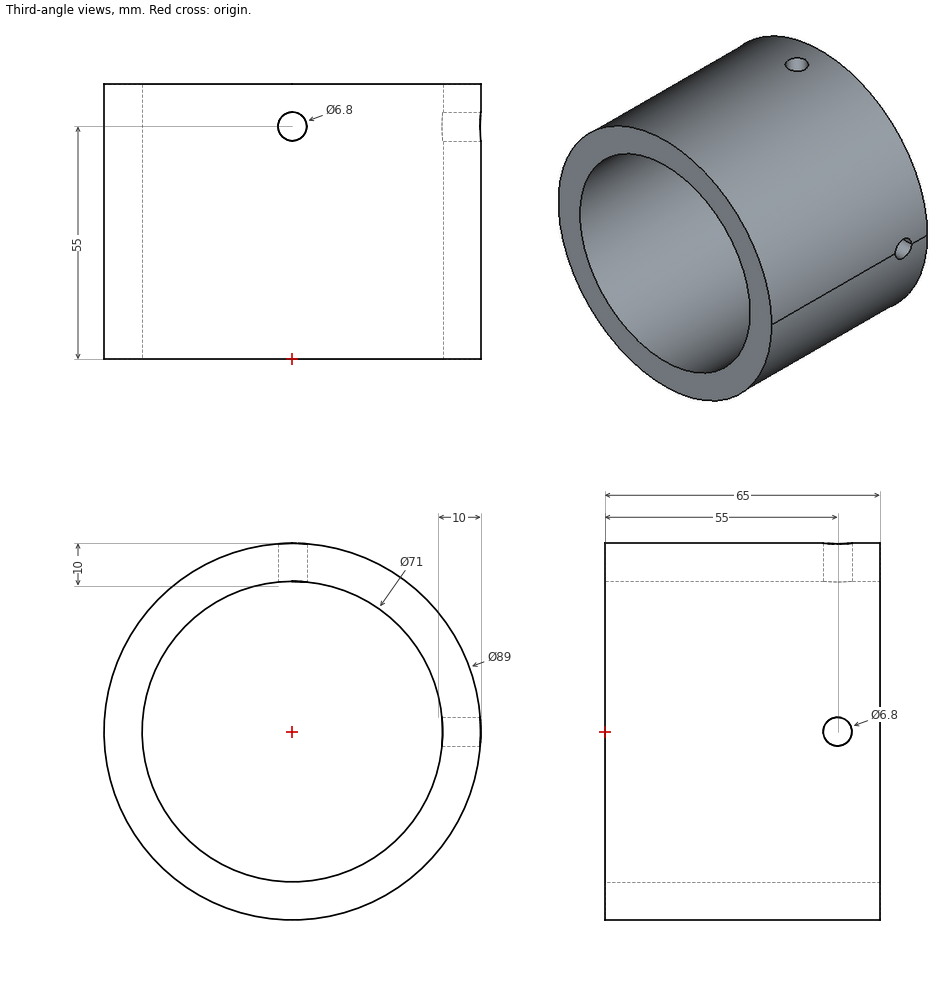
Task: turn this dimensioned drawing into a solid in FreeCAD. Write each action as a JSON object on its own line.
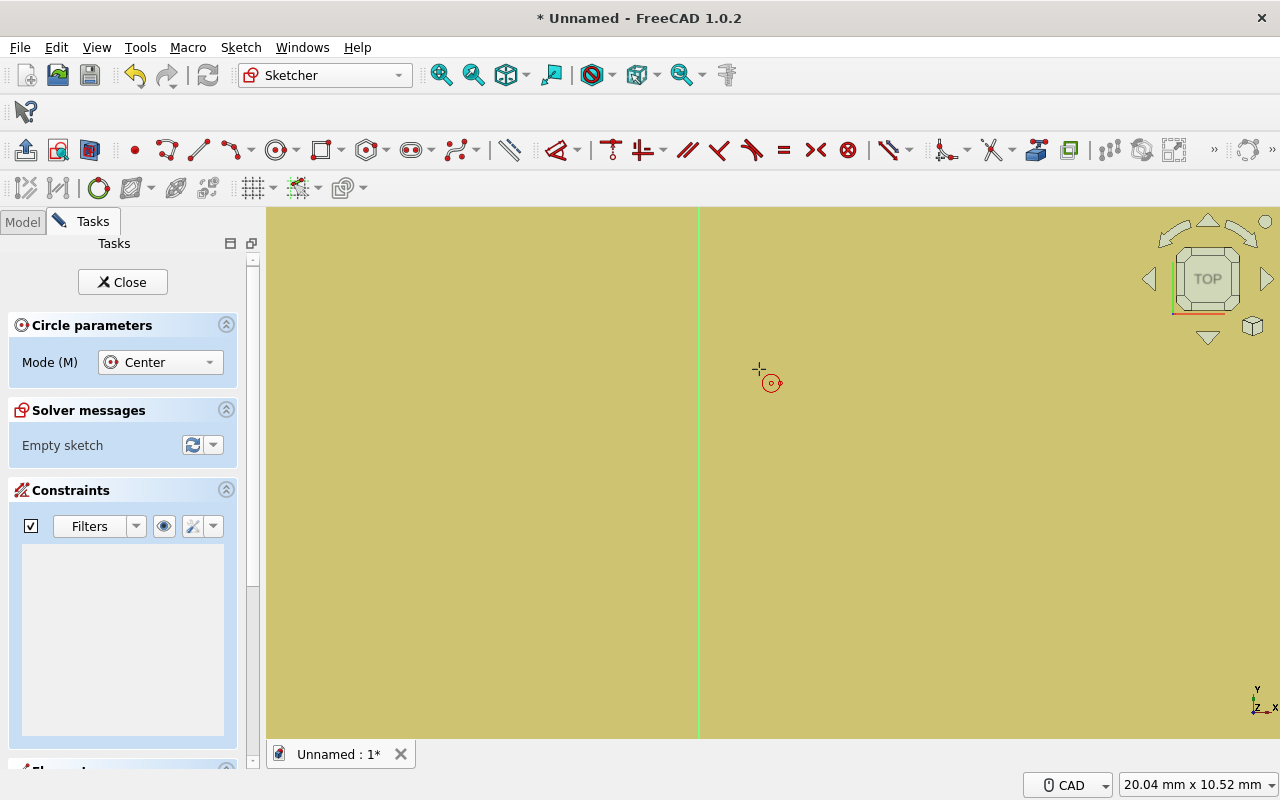
{"action": "left_click", "coordinate": [699, 468]}
{"action": "mouse_move", "coordinate": [821, 347]}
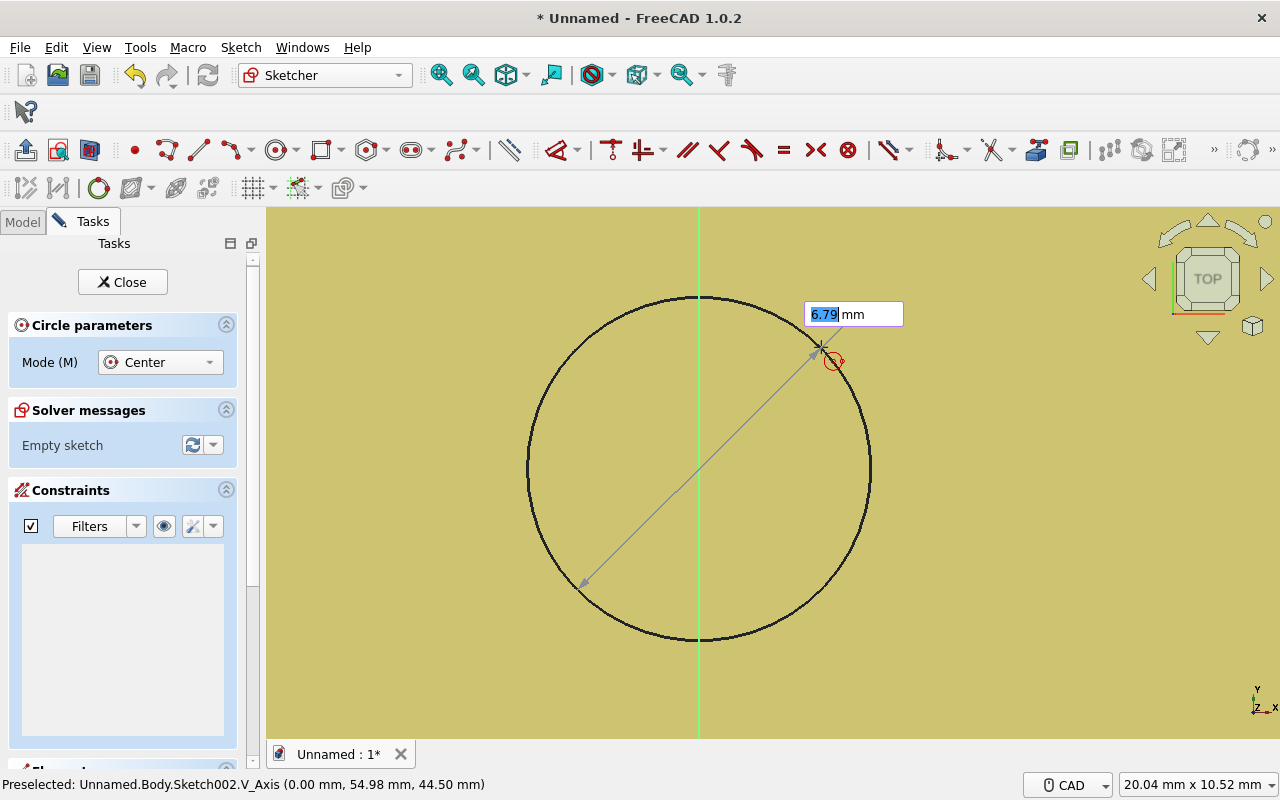
{"action": "type", "text": "6.8"}
{"action": "key", "text": "Return"}
{"action": "key", "text": "Escape"}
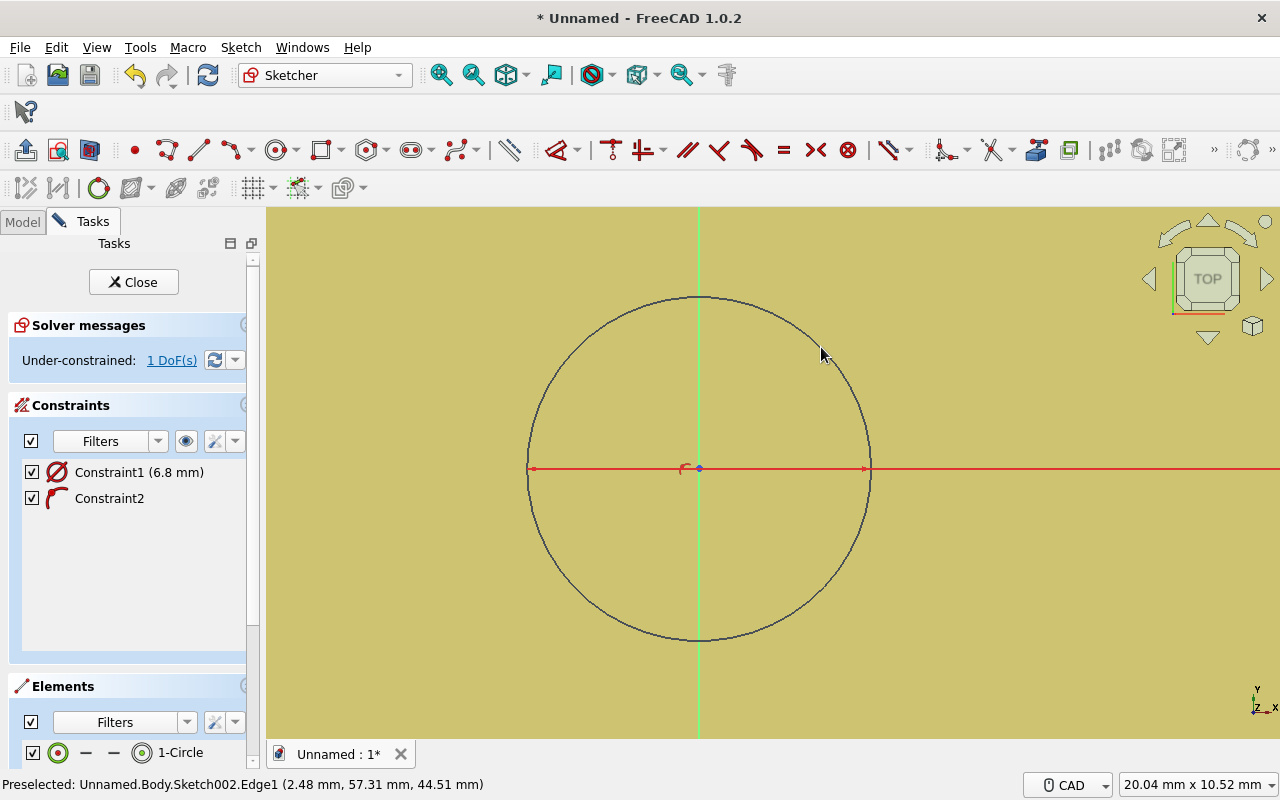
{"action": "key", "text": "d"}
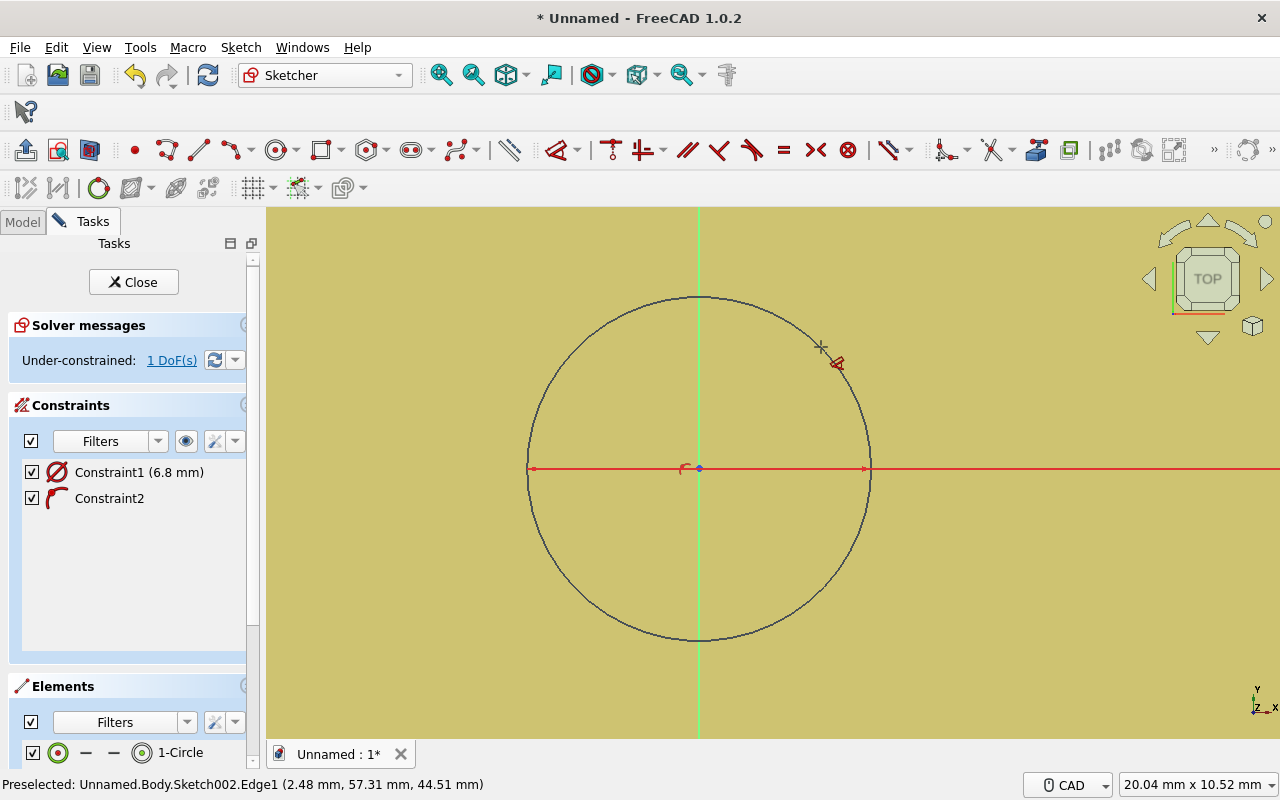
{"action": "left_click", "coordinate": [699, 469]}
{"action": "left_click", "coordinate": [733, 590]}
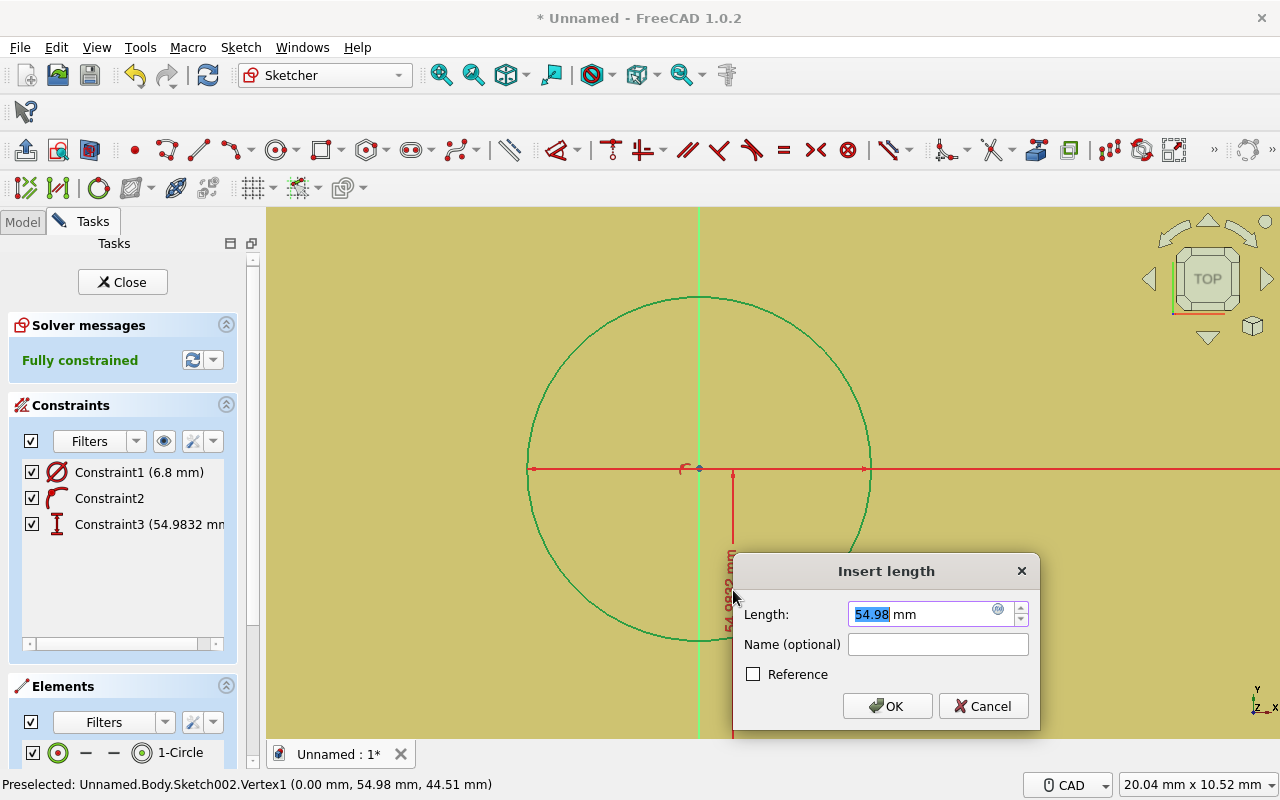
{"action": "type", "text": "55"}
{"action": "key", "text": "Return"}
{"action": "key", "text": "Escape"}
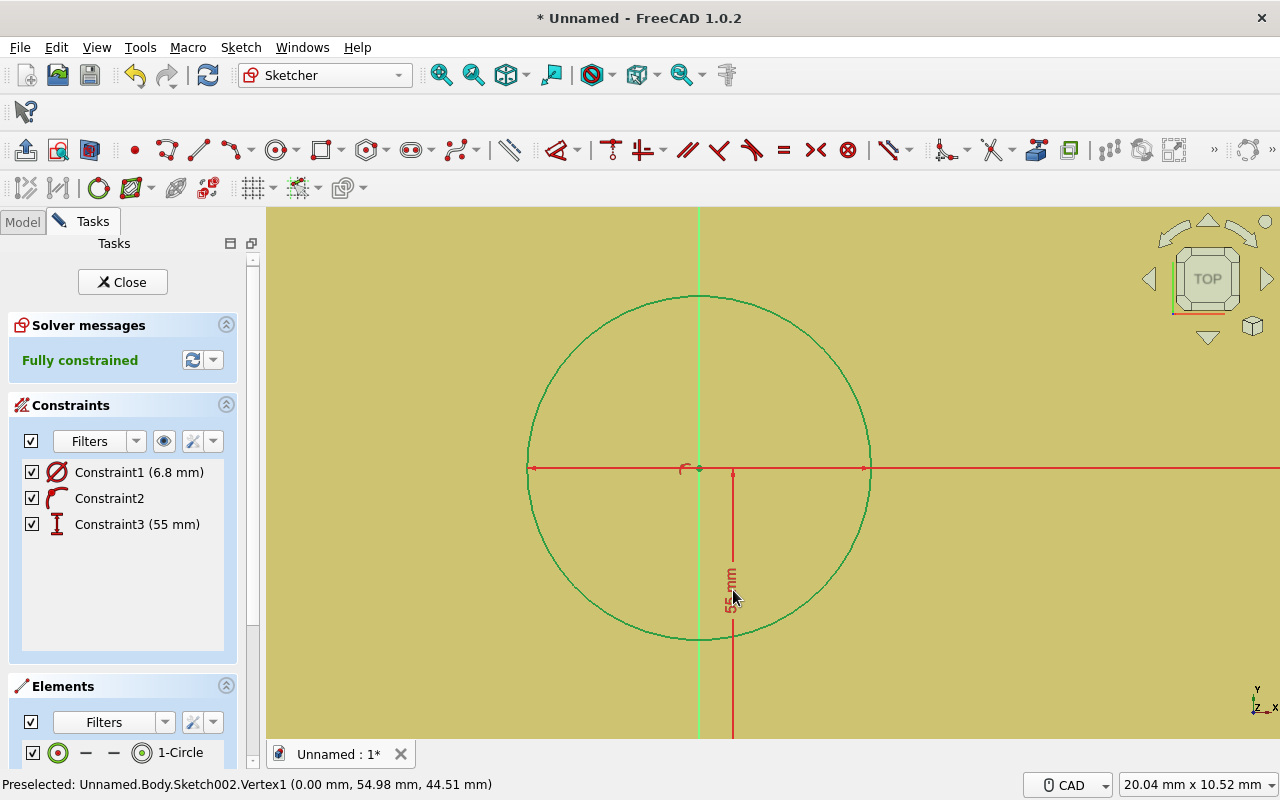
{"action": "left_click", "coordinate": [123, 282]}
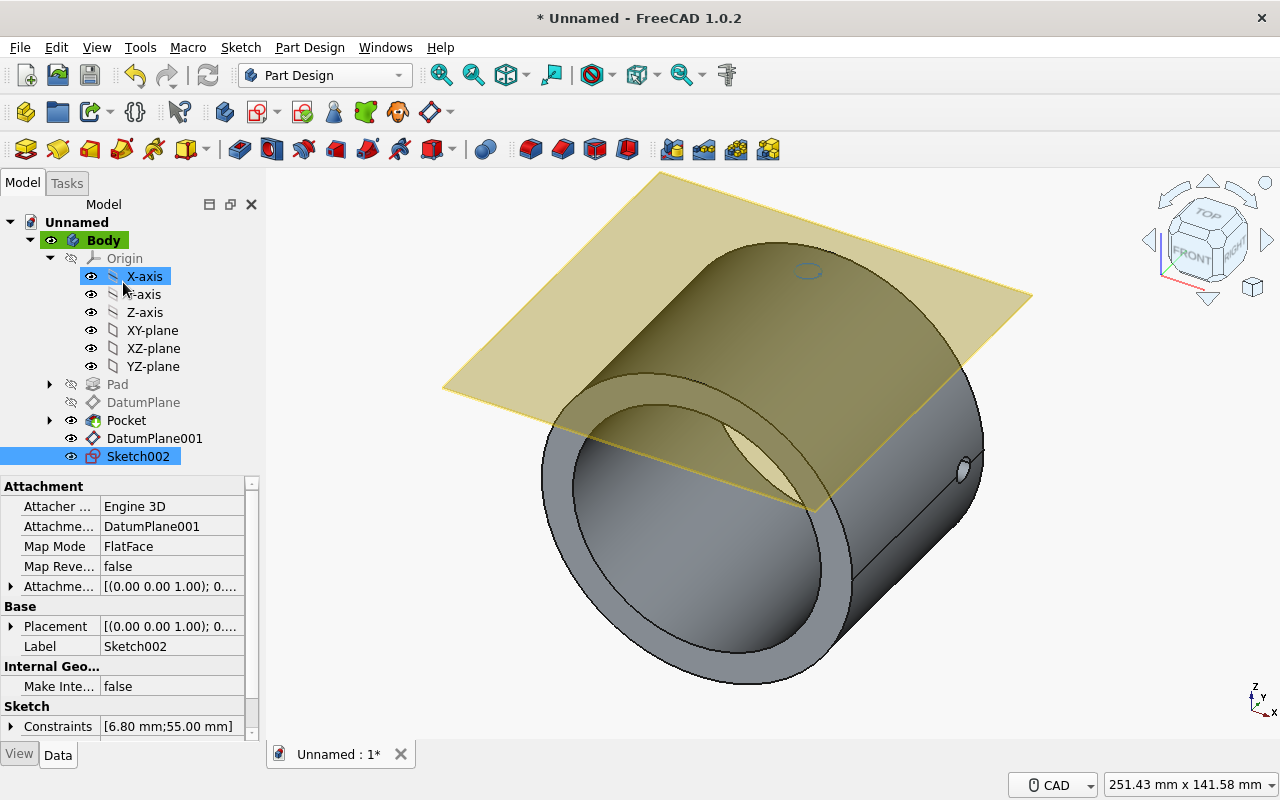
{"action": "left_click", "coordinate": [240, 150]}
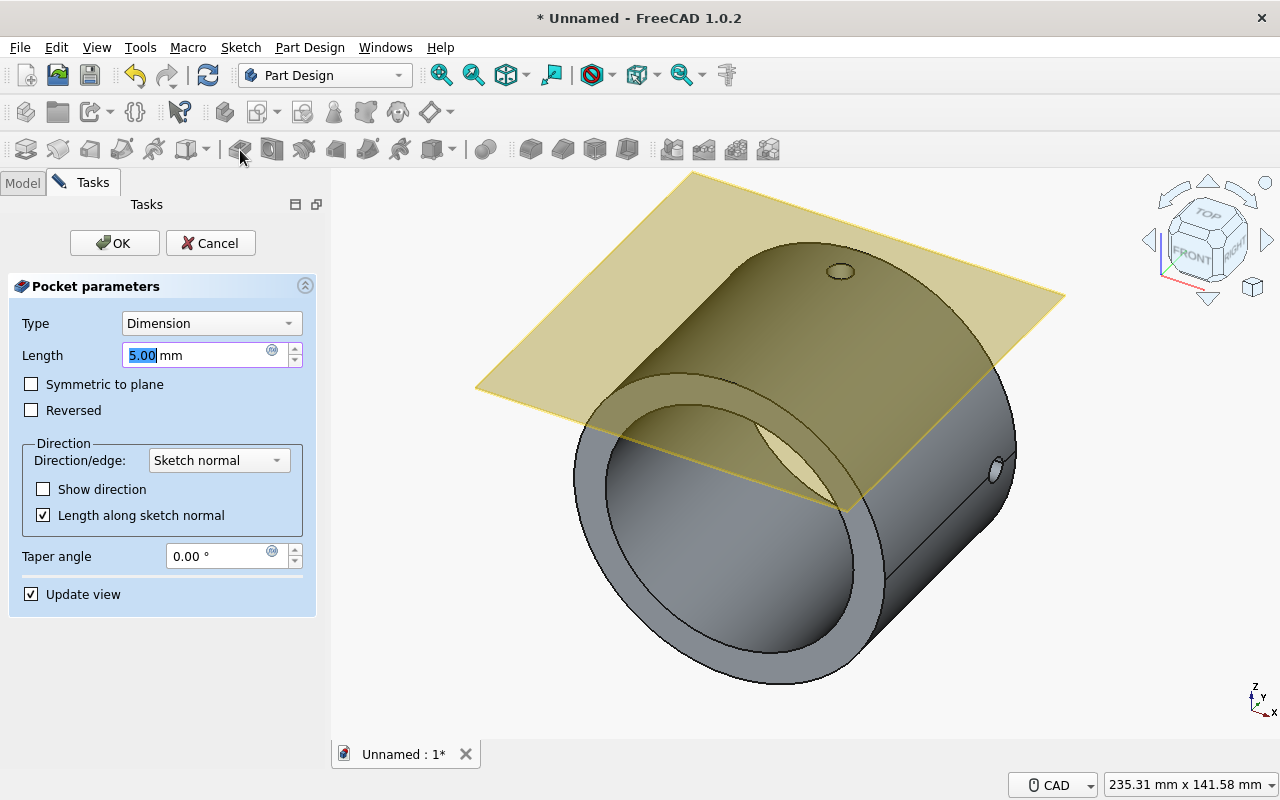
{"action": "type", "text": "10"}
{"action": "key", "text": "Tab"}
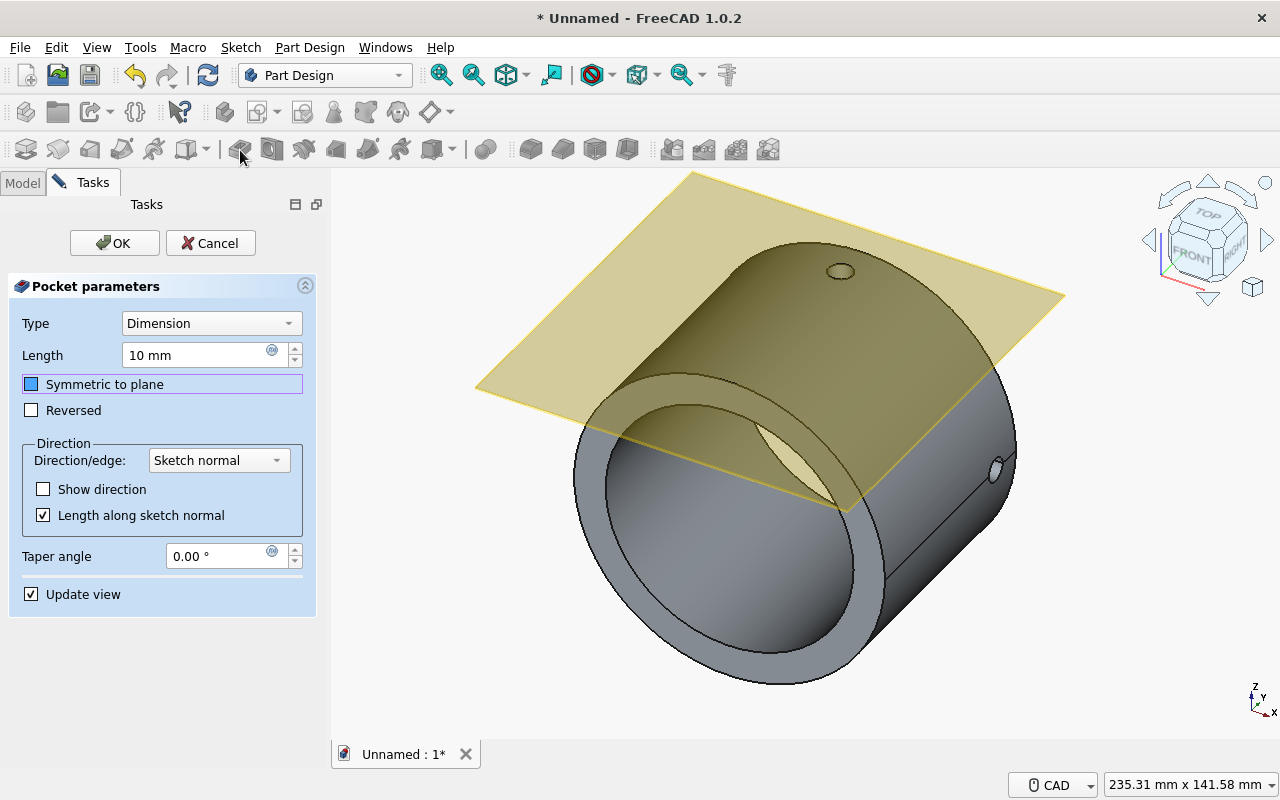
{"action": "left_click", "coordinate": [115, 243]}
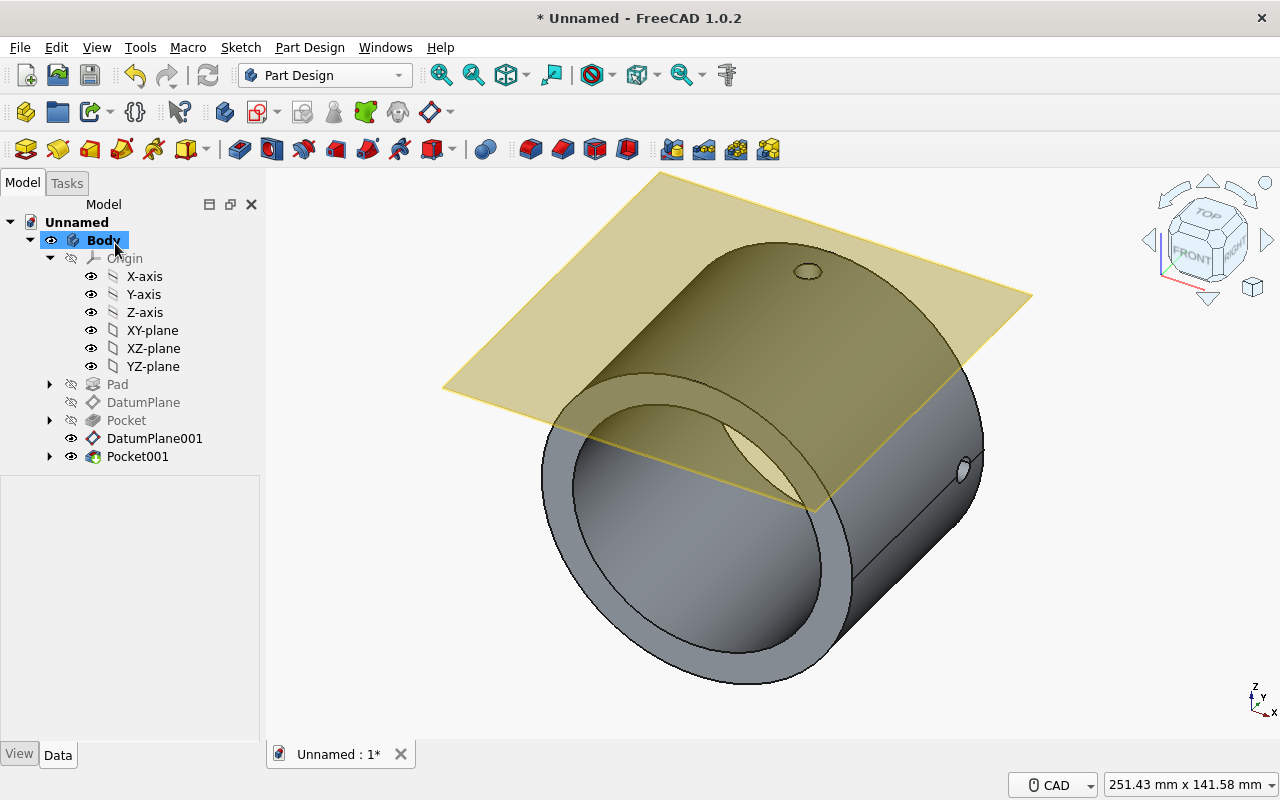
{"action": "left_click", "coordinate": [116, 438]}
{"action": "key", "text": "space"}